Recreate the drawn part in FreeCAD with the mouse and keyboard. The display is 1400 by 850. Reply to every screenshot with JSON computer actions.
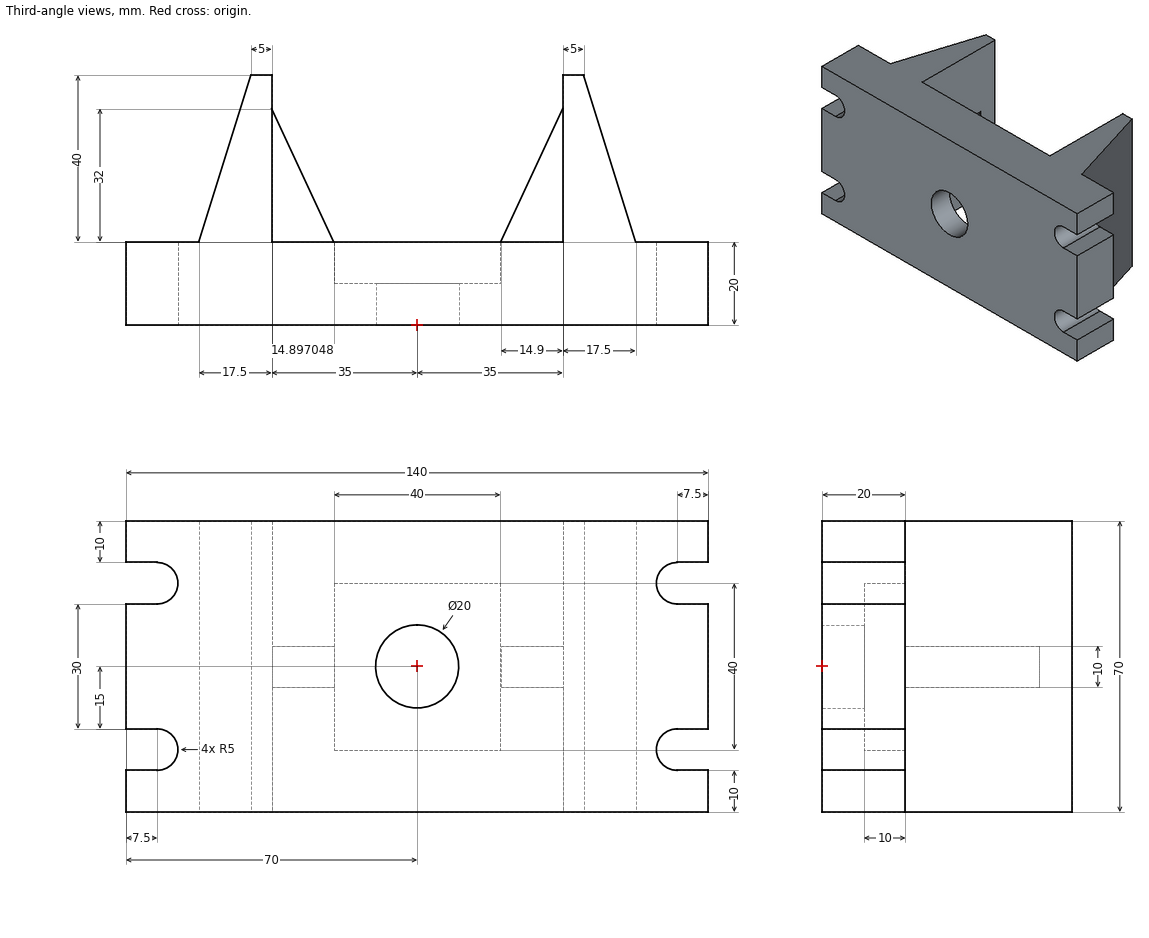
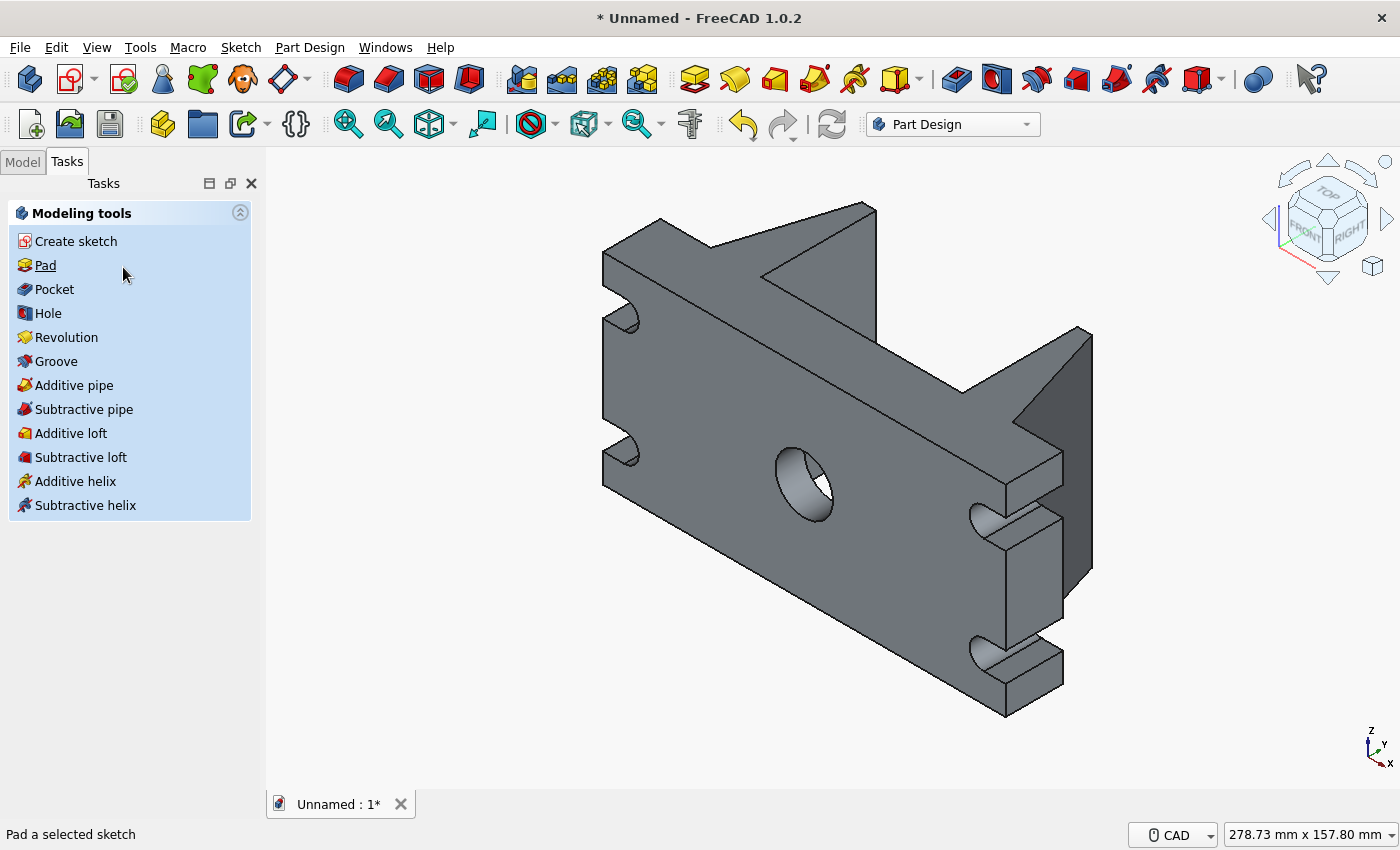
{"action": "left_click", "coordinate": [696, 80]}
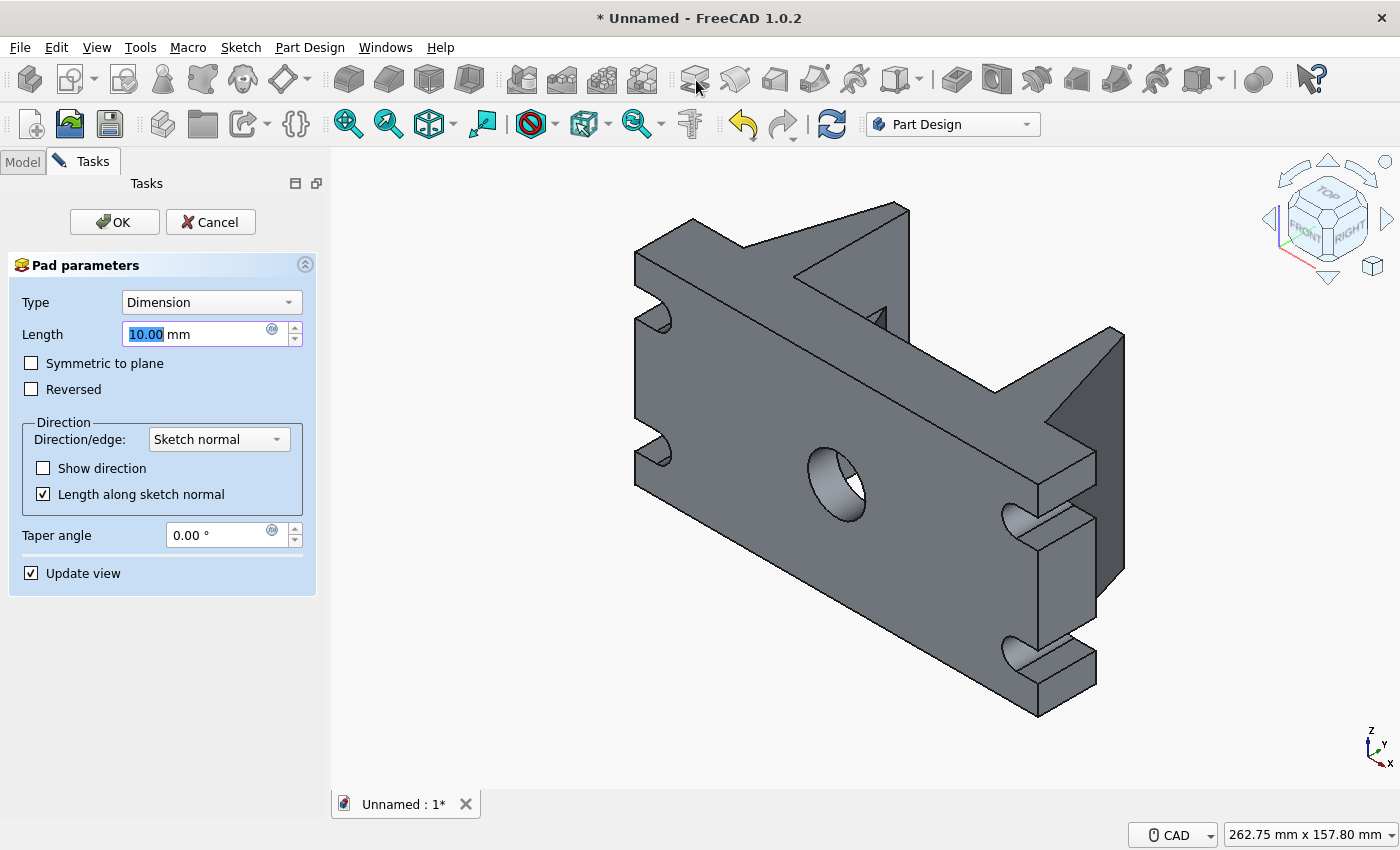
{"action": "type", "text": "10"}
{"action": "key", "text": "Tab"}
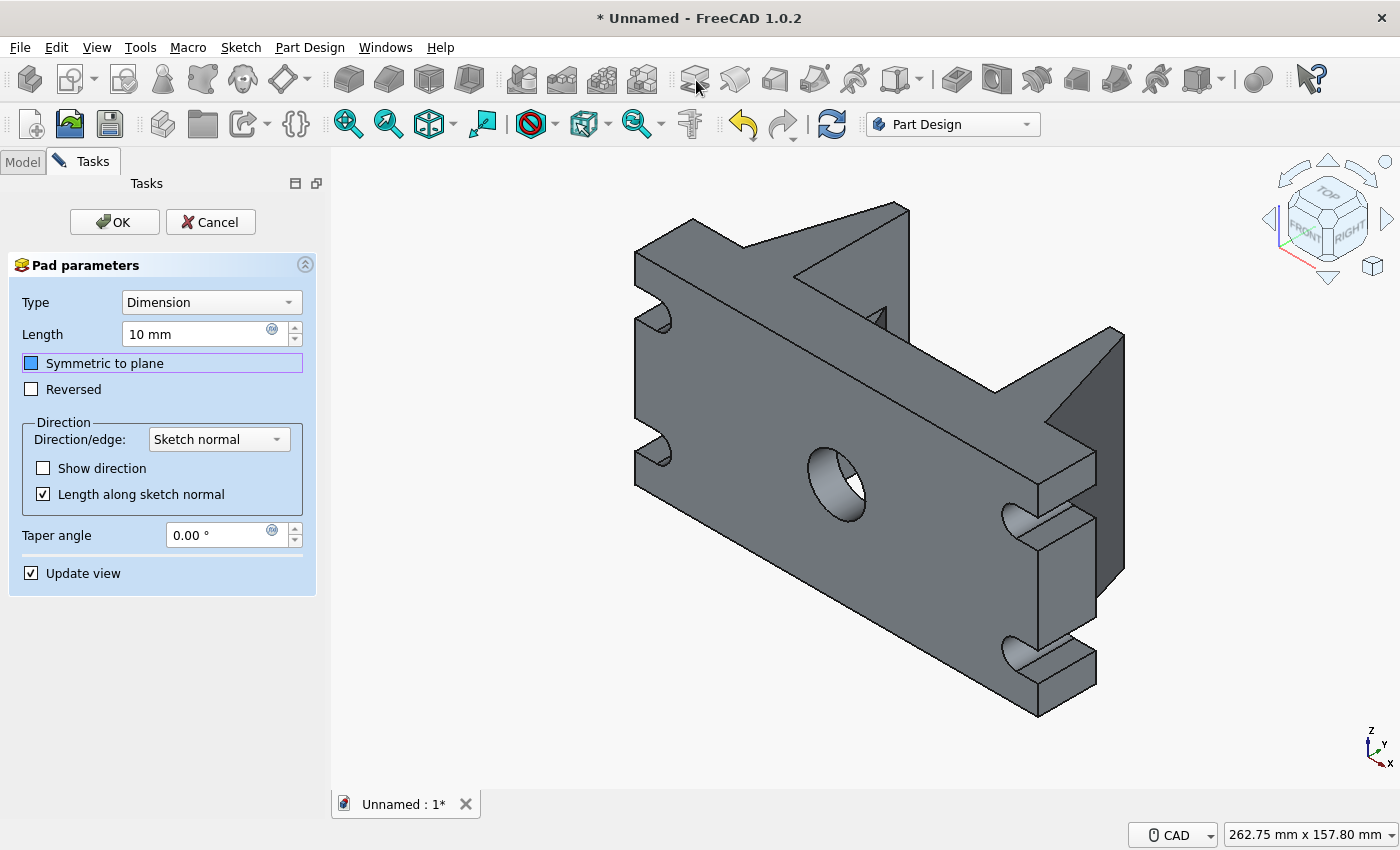
{"action": "left_click", "coordinate": [30, 363]}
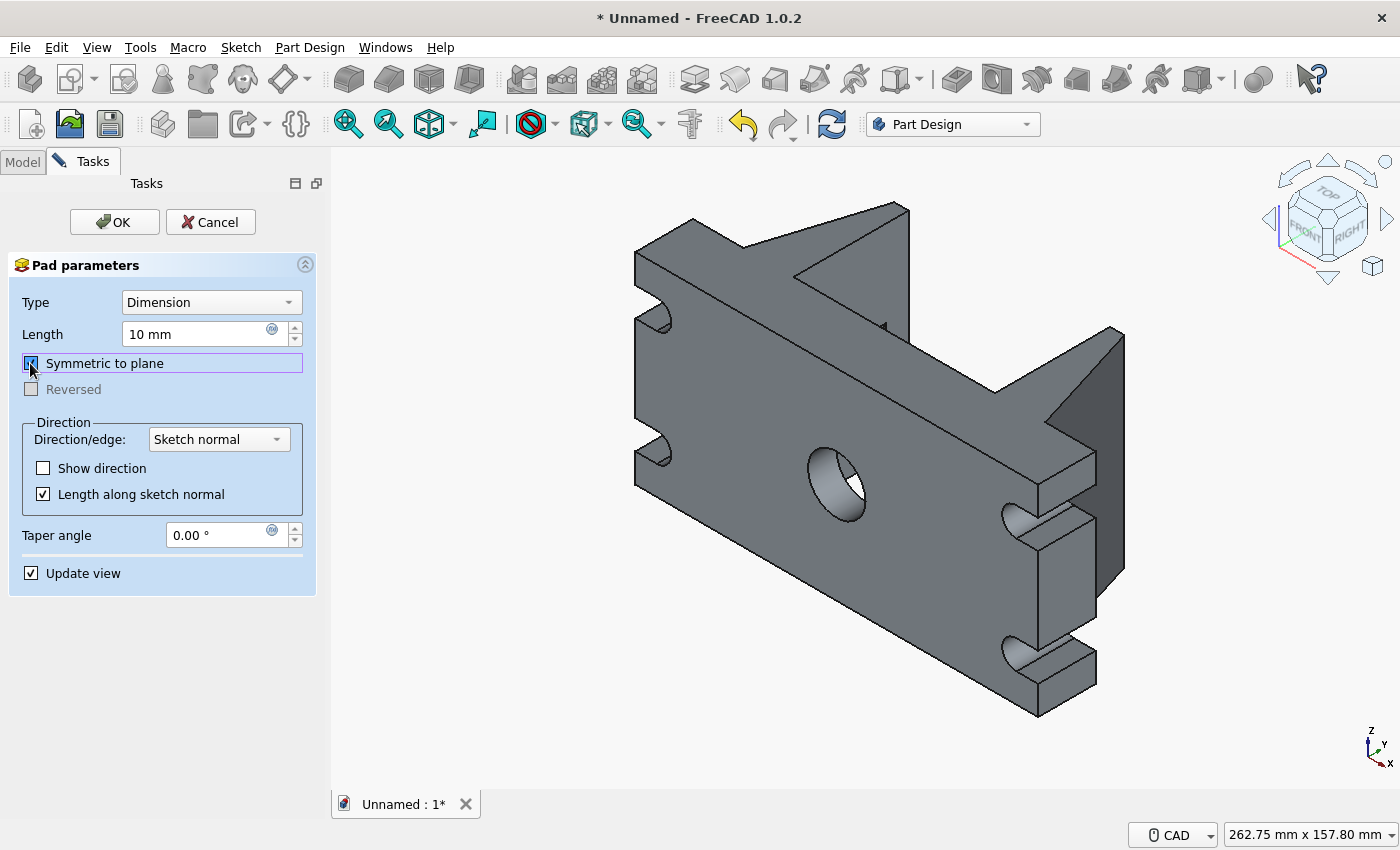
{"action": "left_click", "coordinate": [115, 222]}